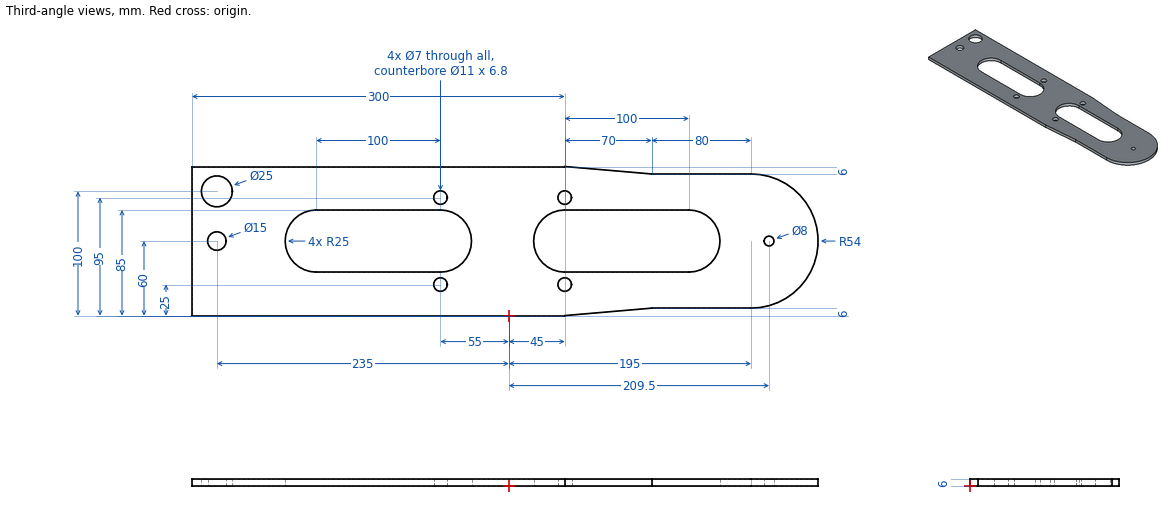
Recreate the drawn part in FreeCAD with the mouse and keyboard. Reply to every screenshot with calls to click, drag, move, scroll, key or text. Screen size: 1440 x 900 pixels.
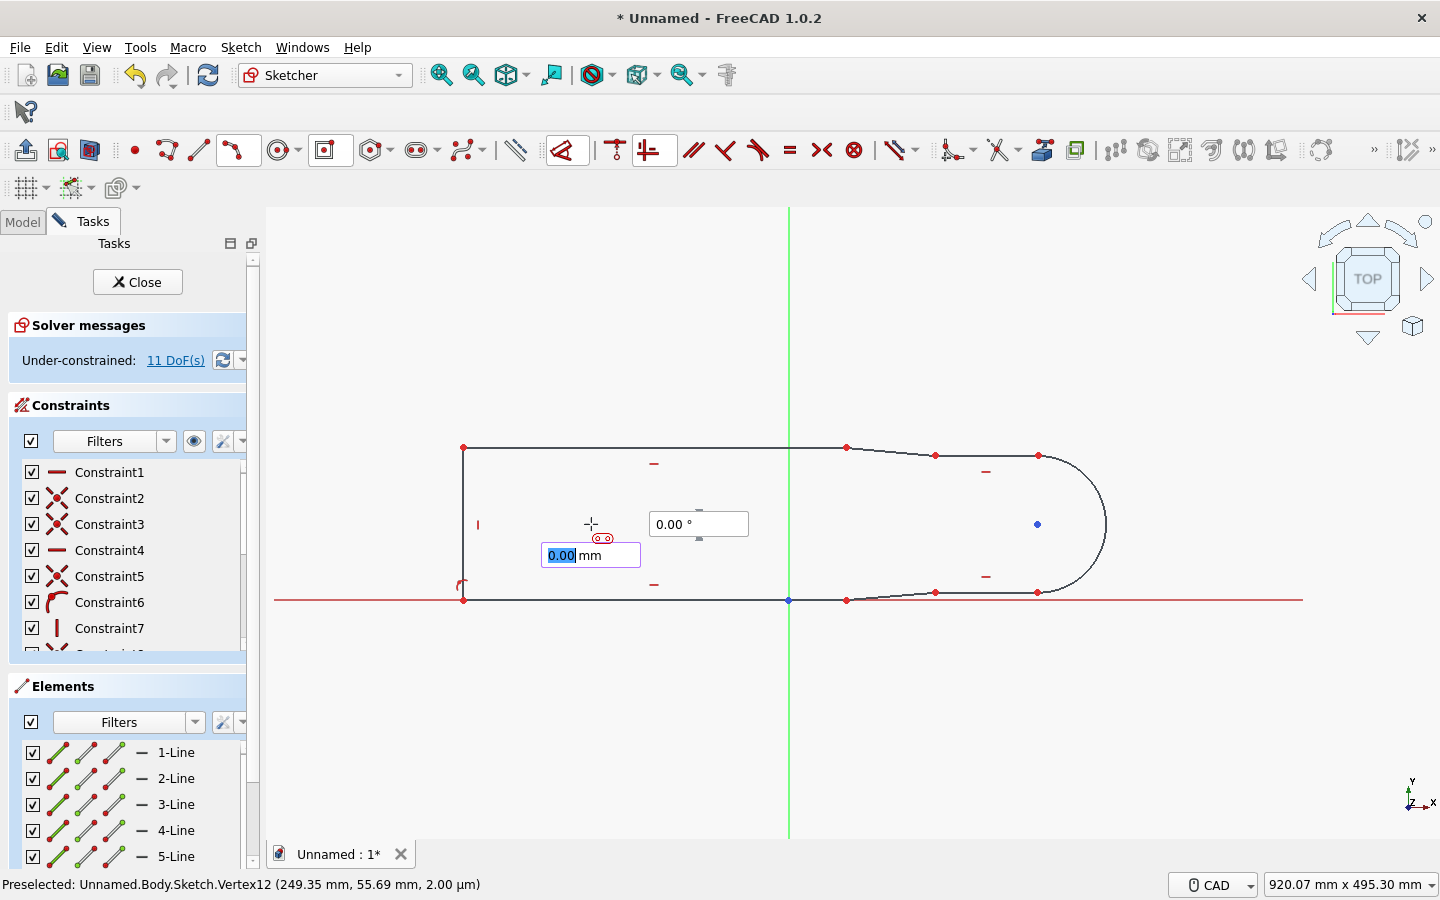
click(719, 524)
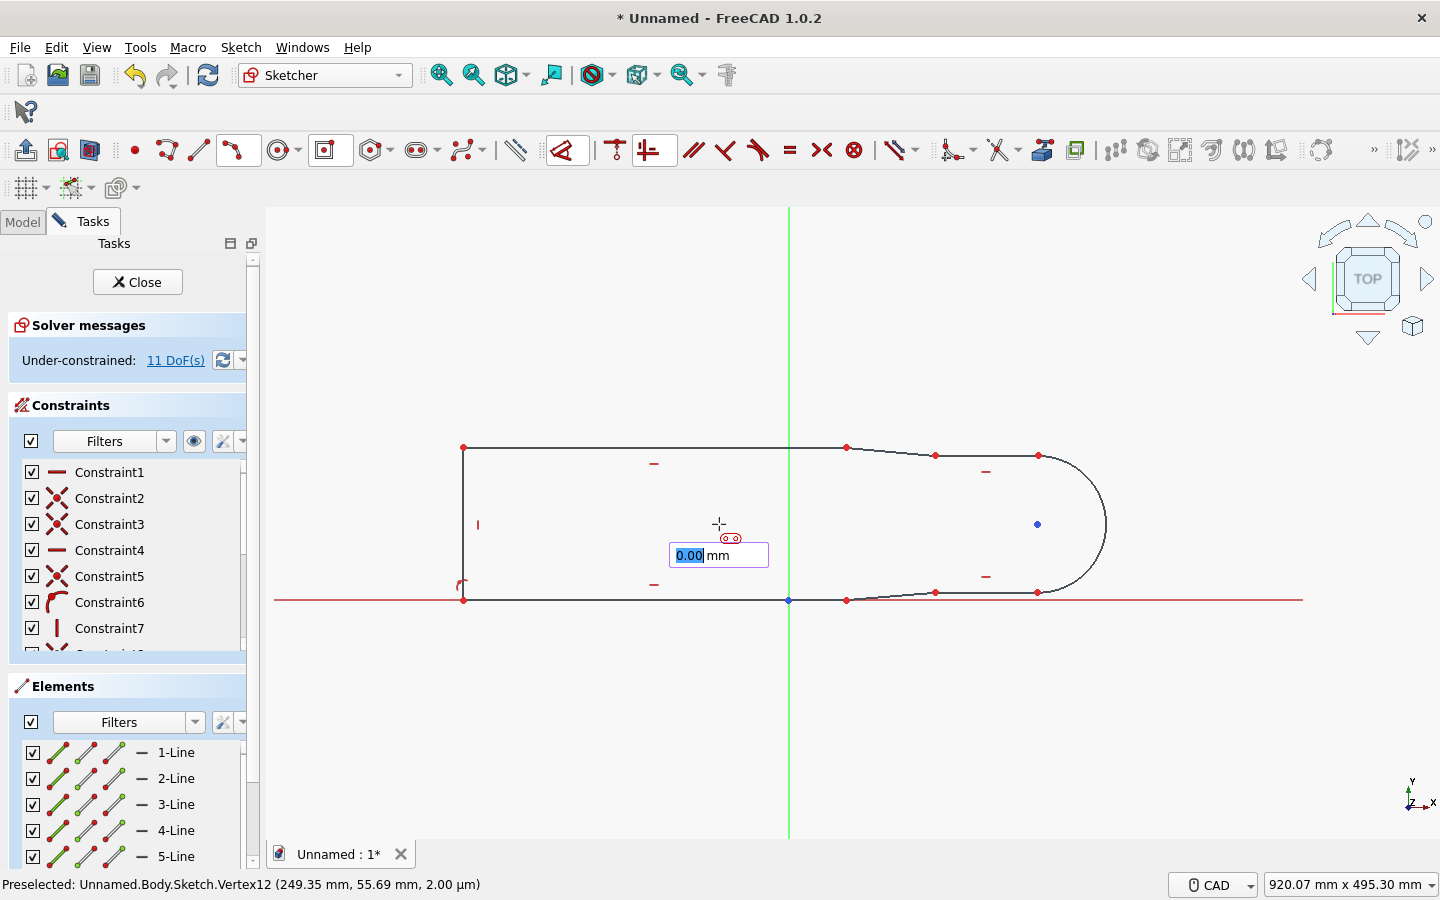
click(655, 492)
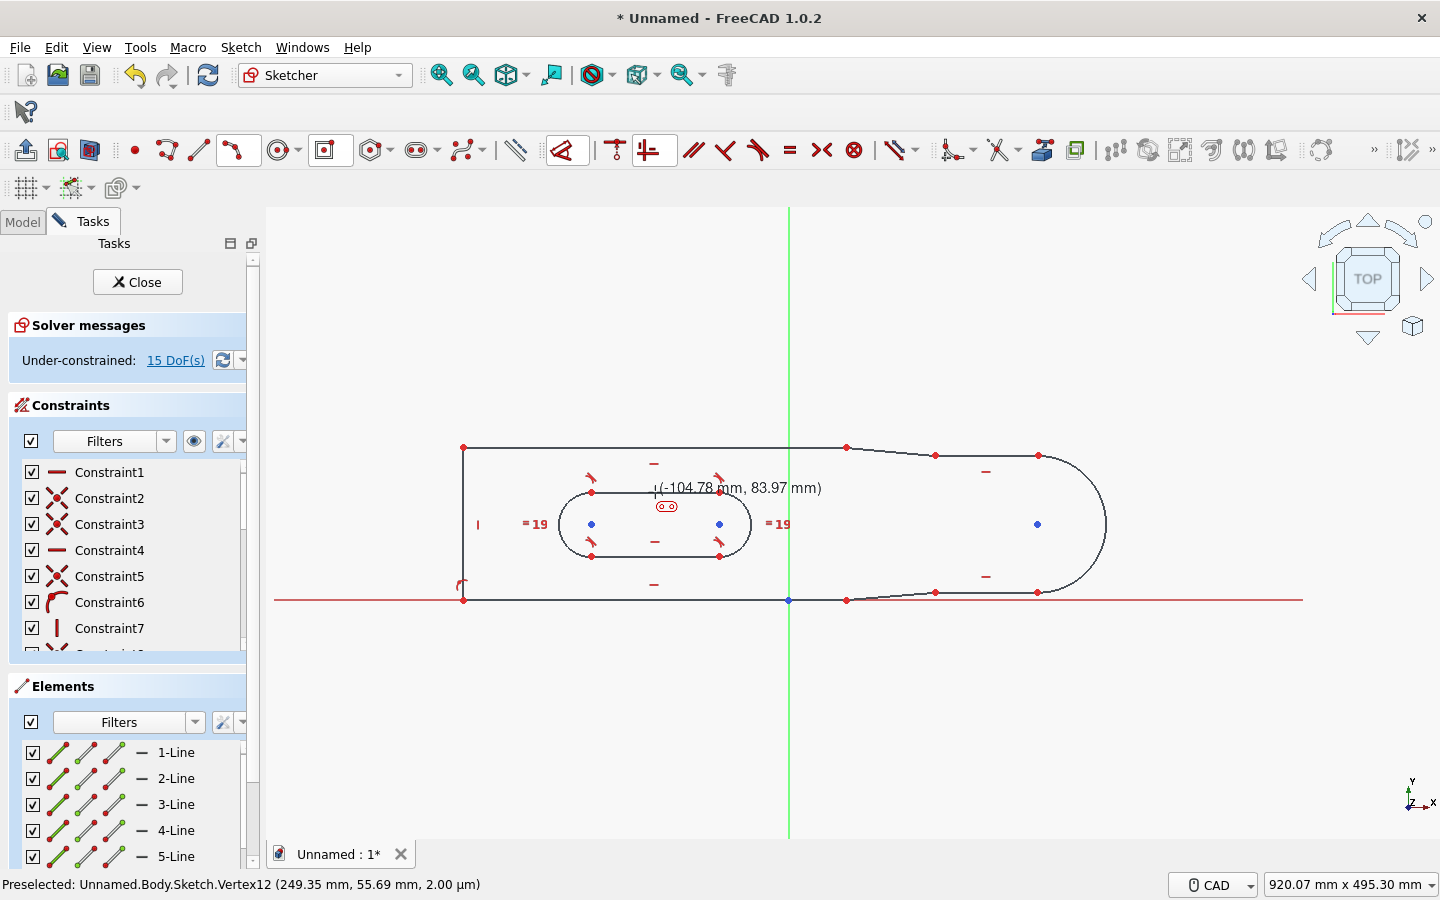
click(846, 524)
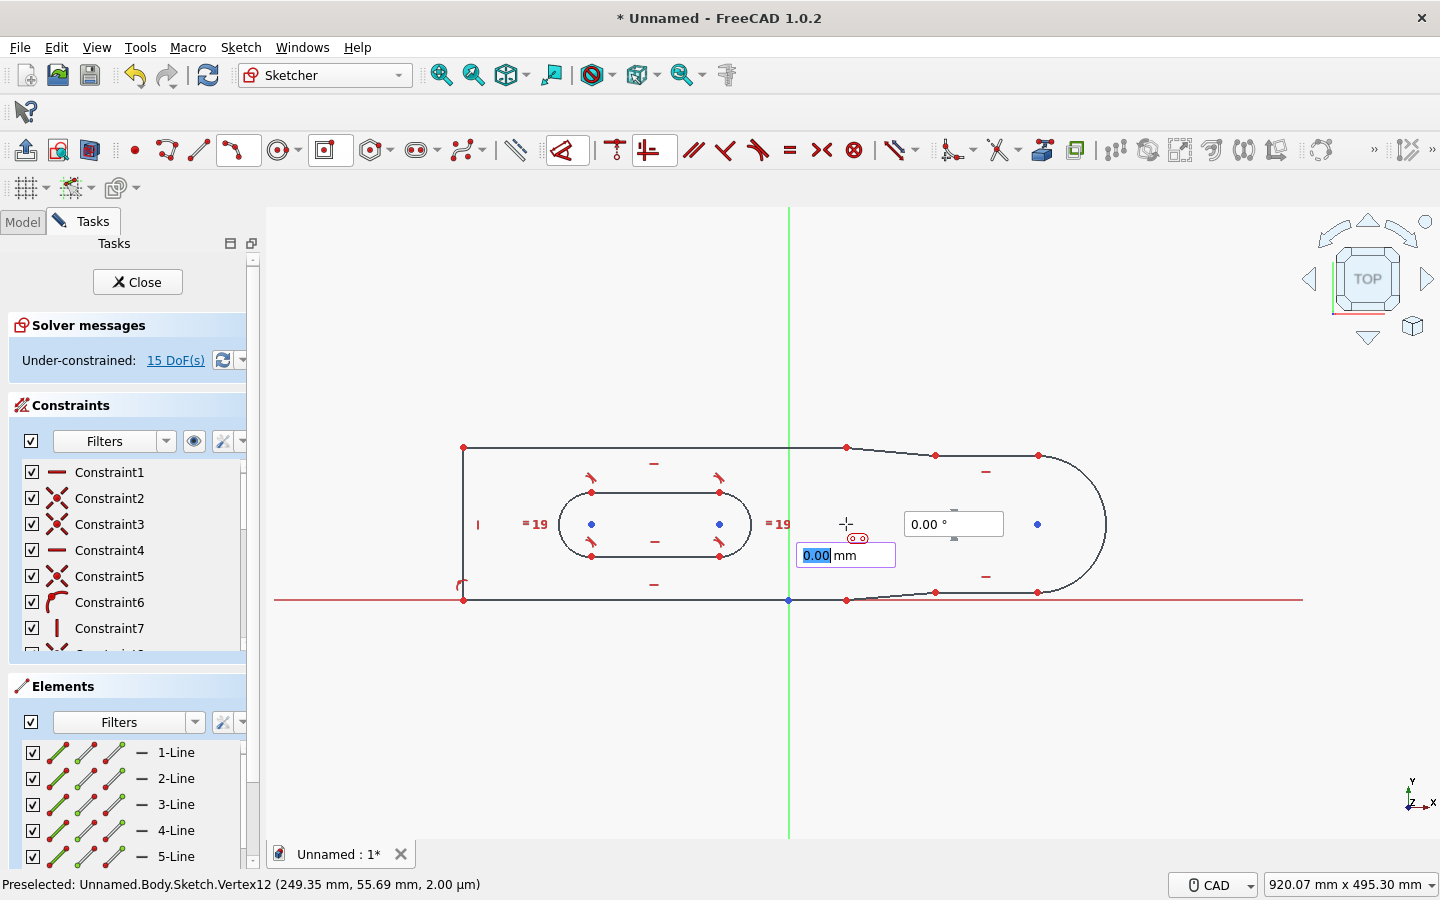
click(974, 524)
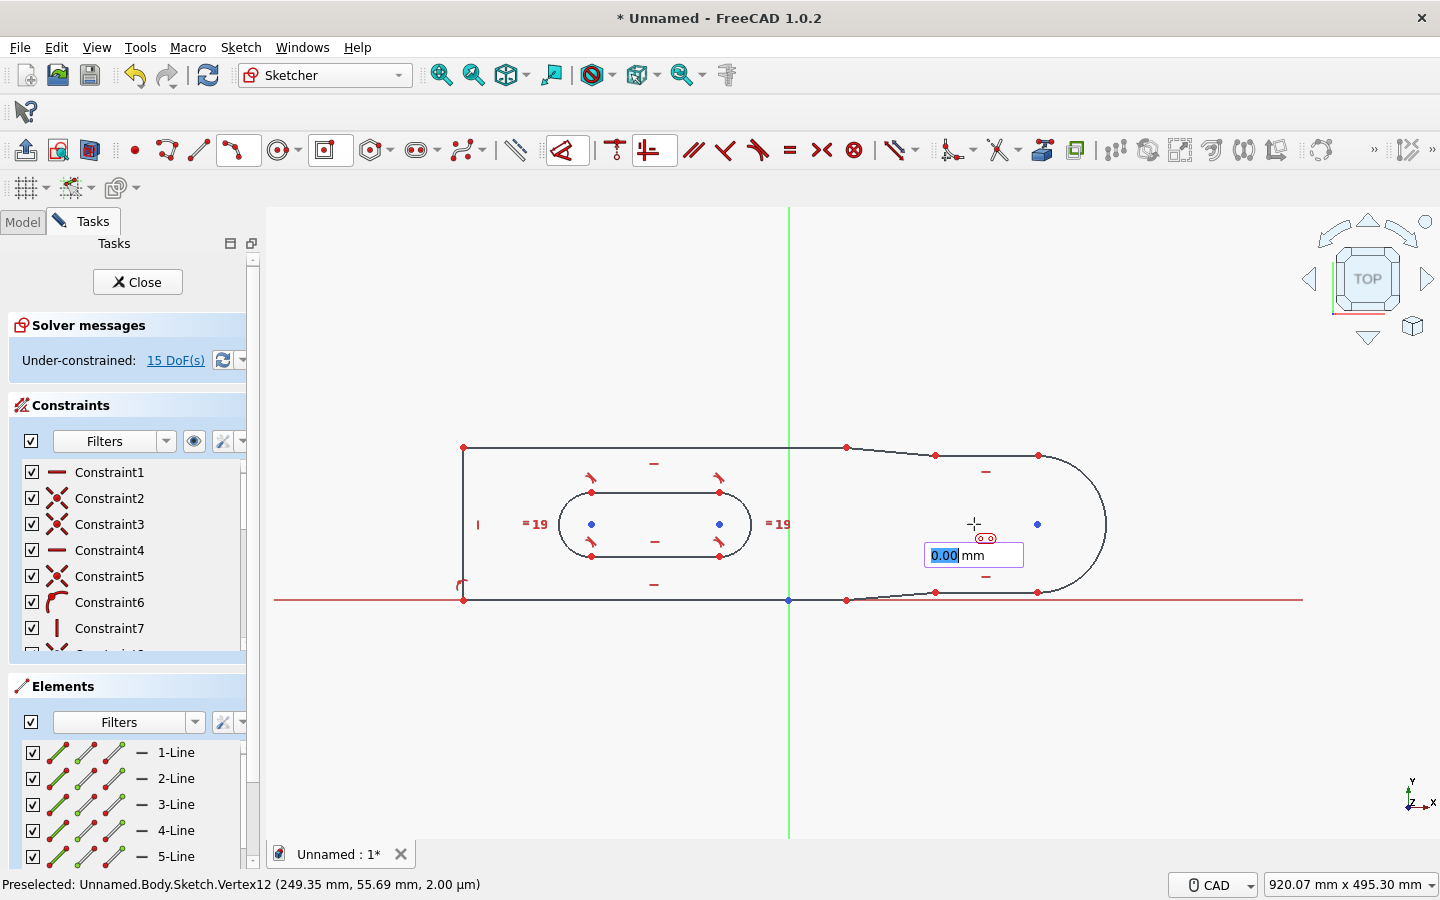
click(910, 492)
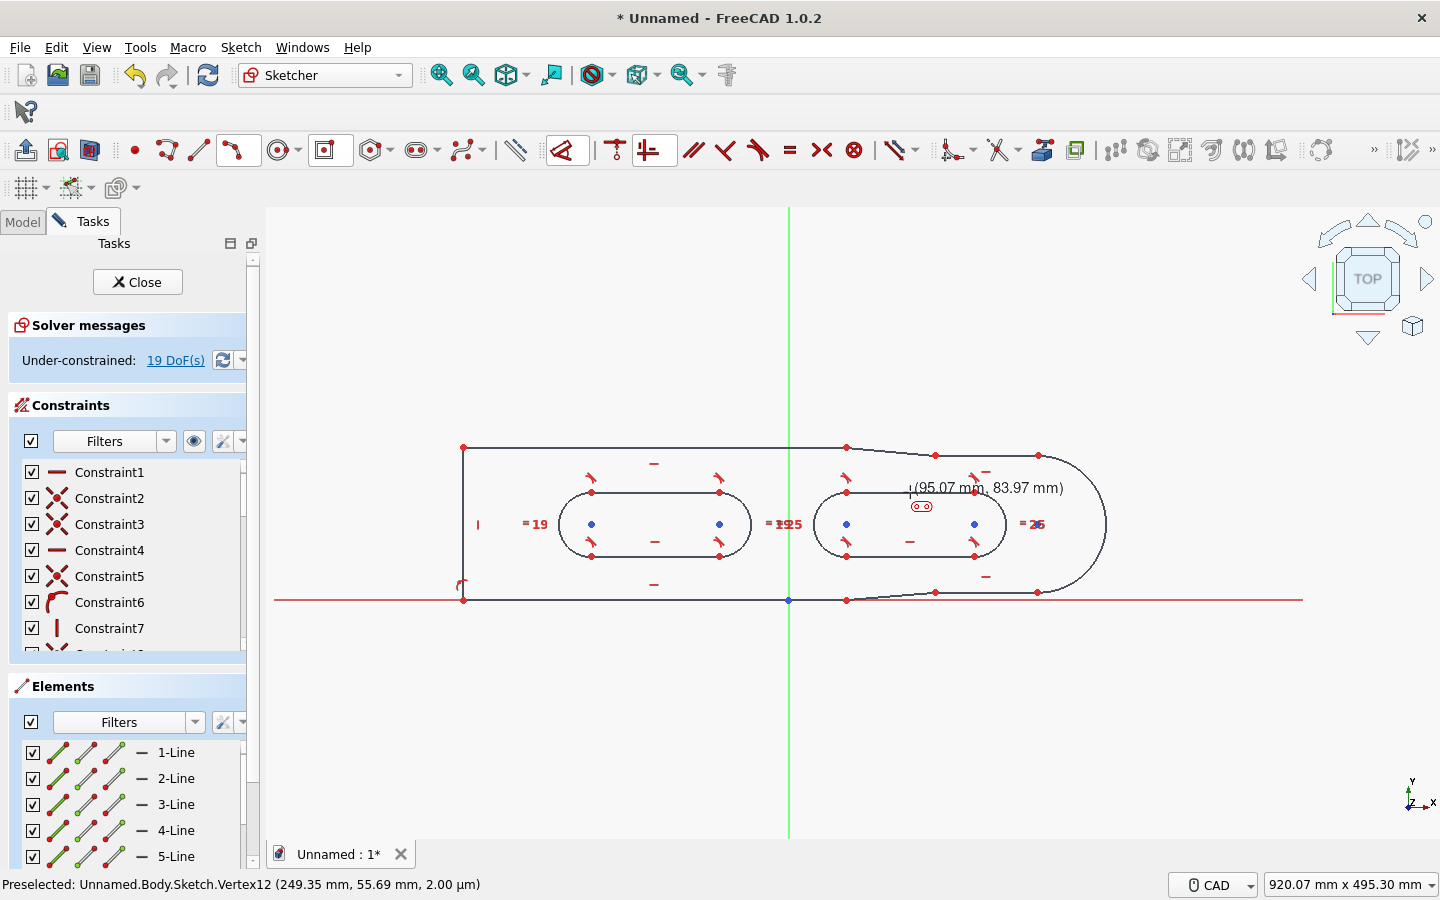
key(g)
key(c)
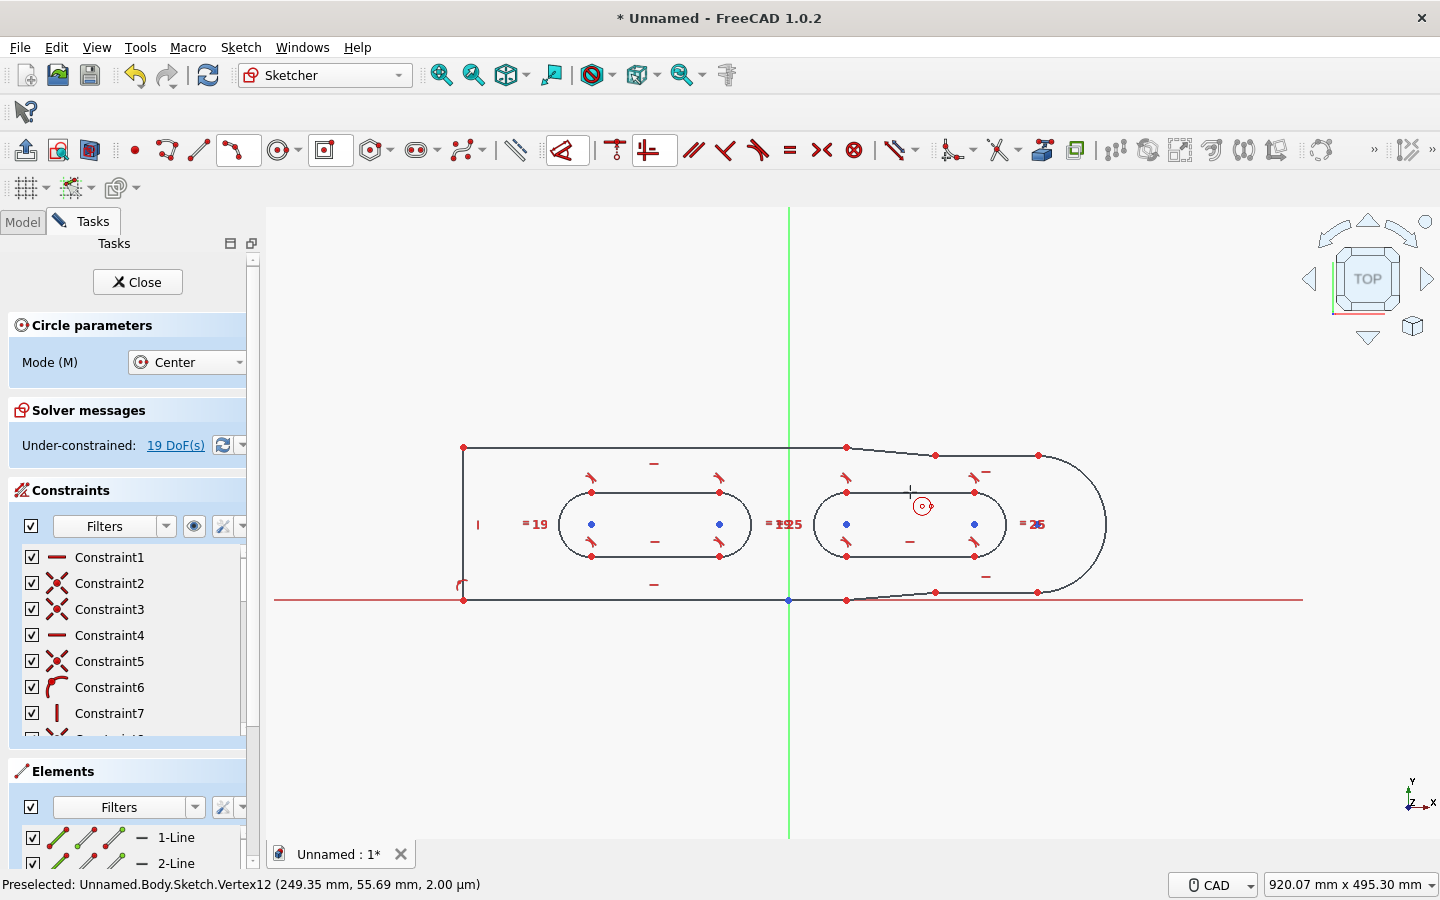
scroll(489, 524, up, 5)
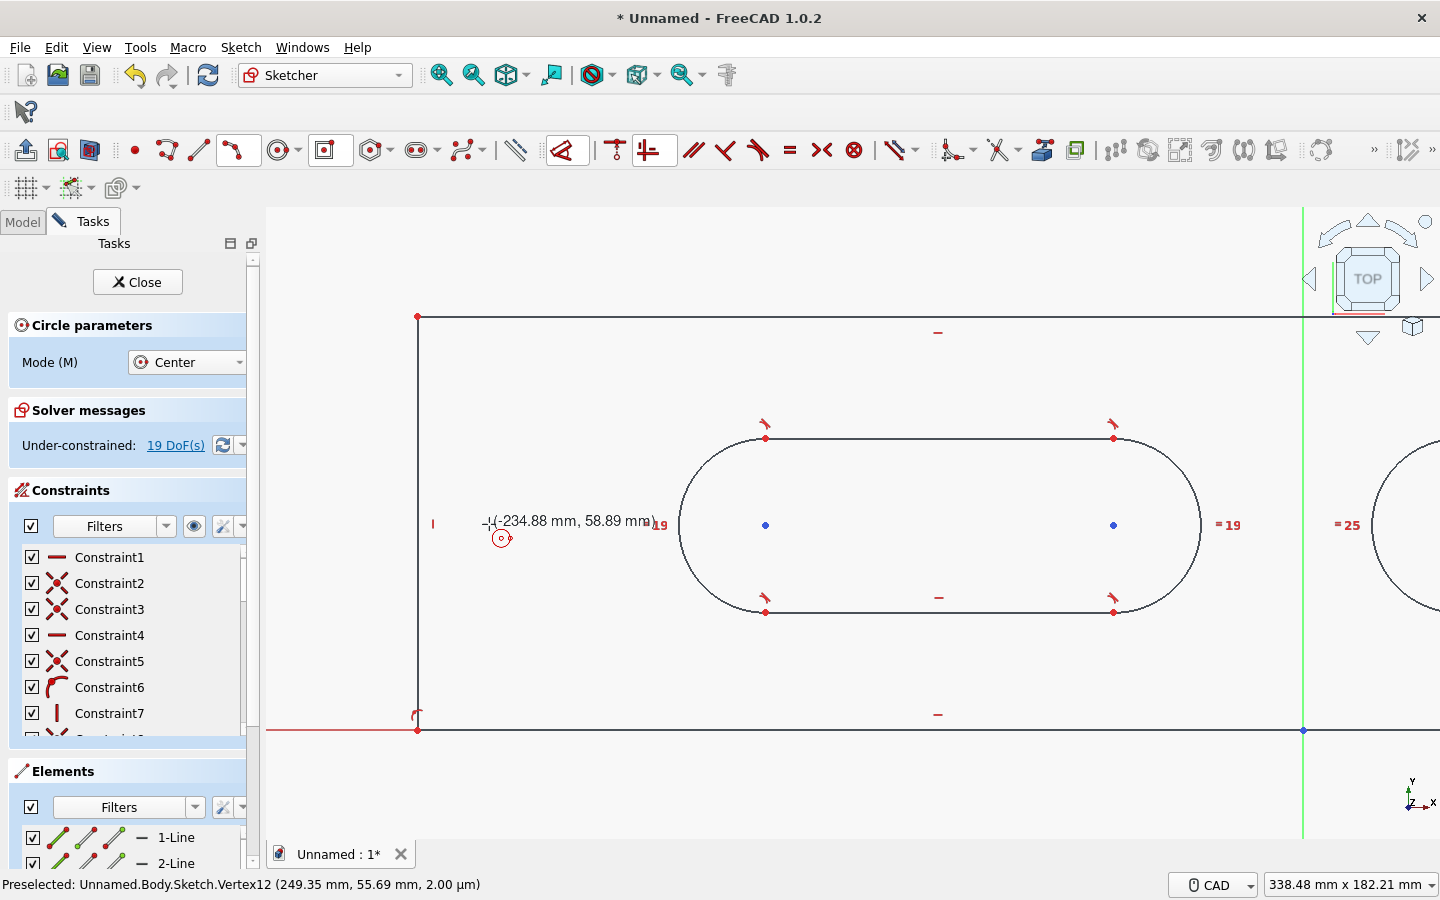
click(488, 522)
move(507, 504)